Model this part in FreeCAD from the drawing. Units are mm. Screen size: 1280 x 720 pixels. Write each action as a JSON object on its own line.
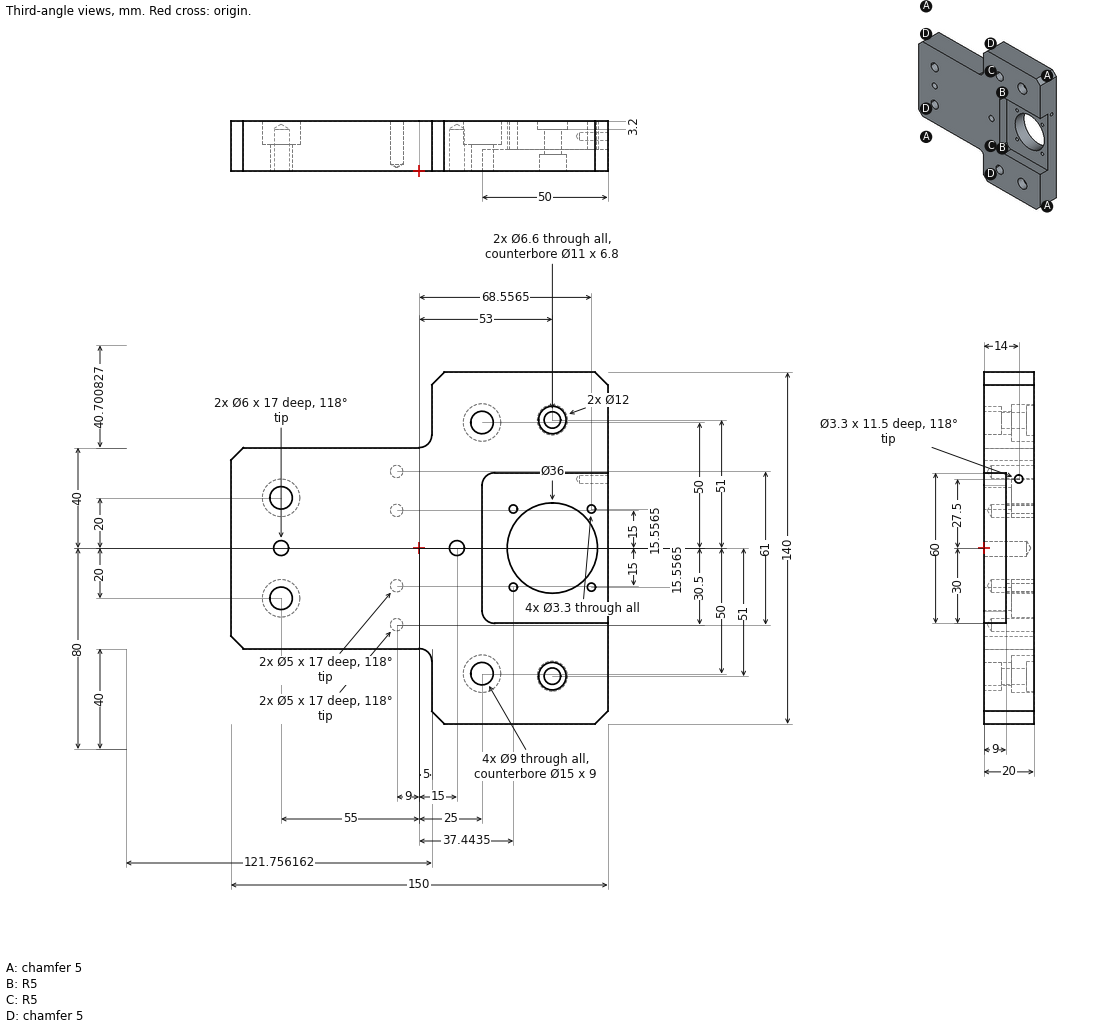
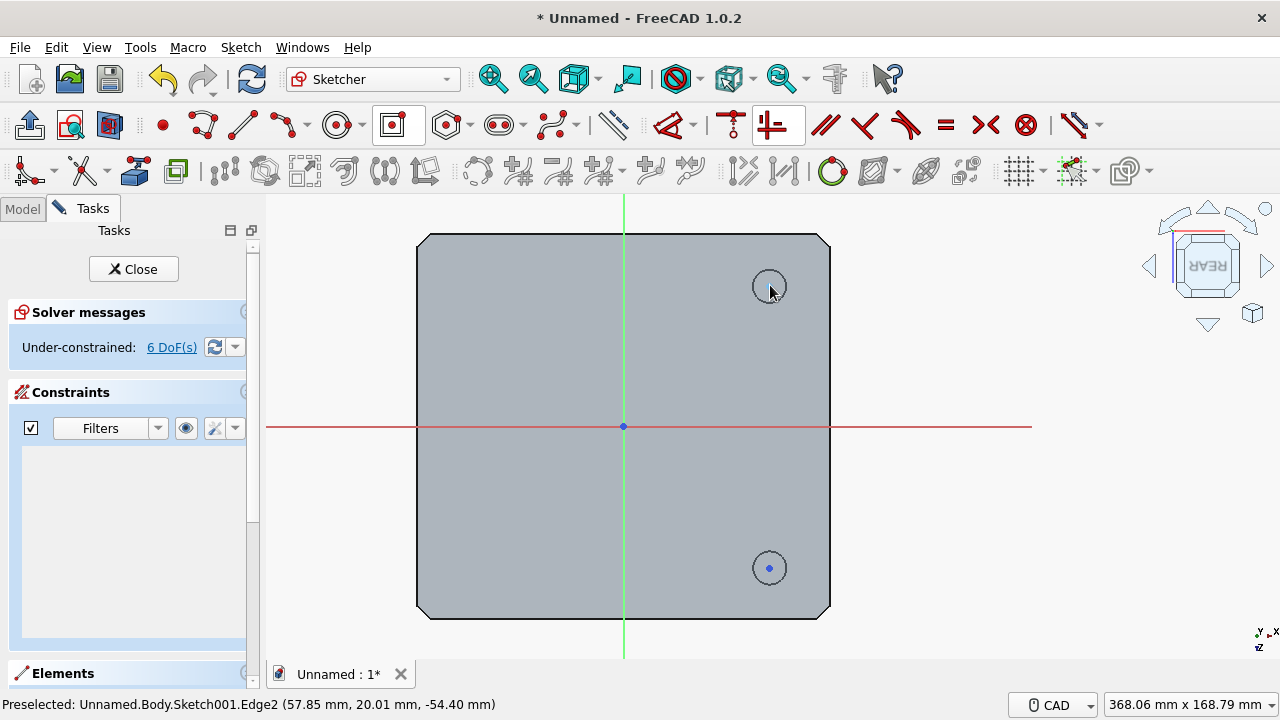
{"action": "left_click", "coordinate": [781, 556]}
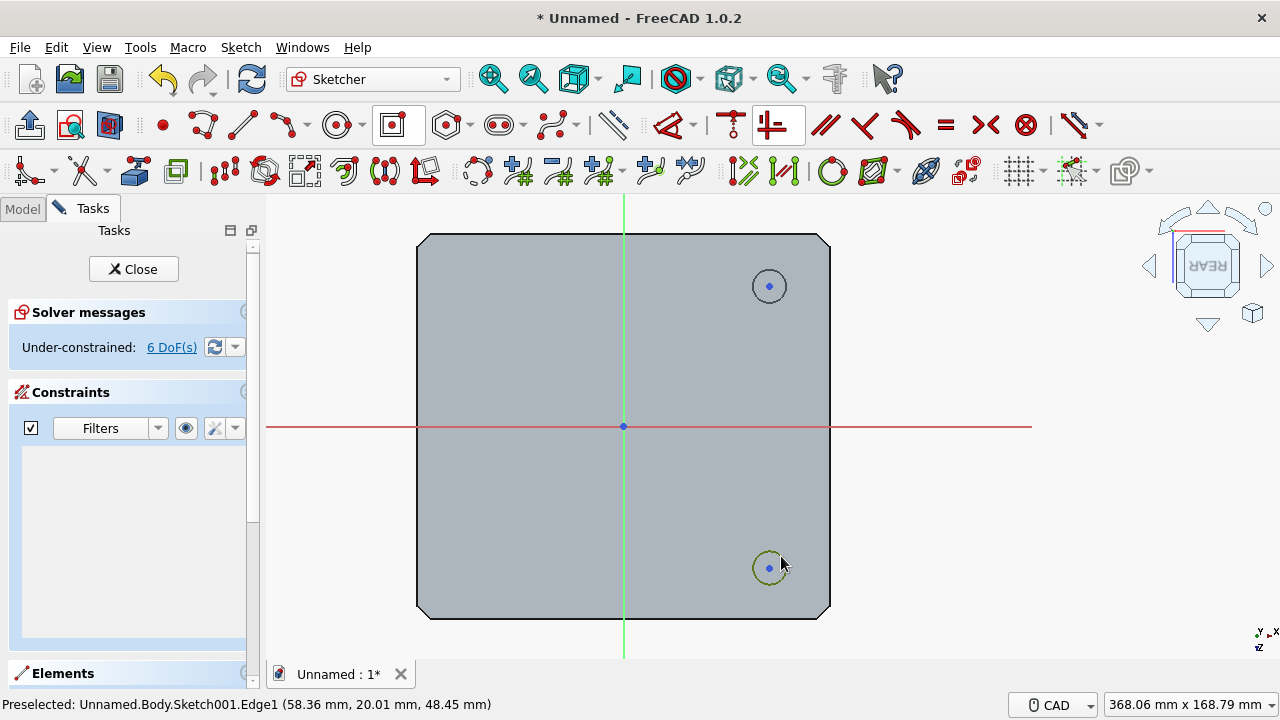
{"action": "left_click", "coordinate": [781, 275]}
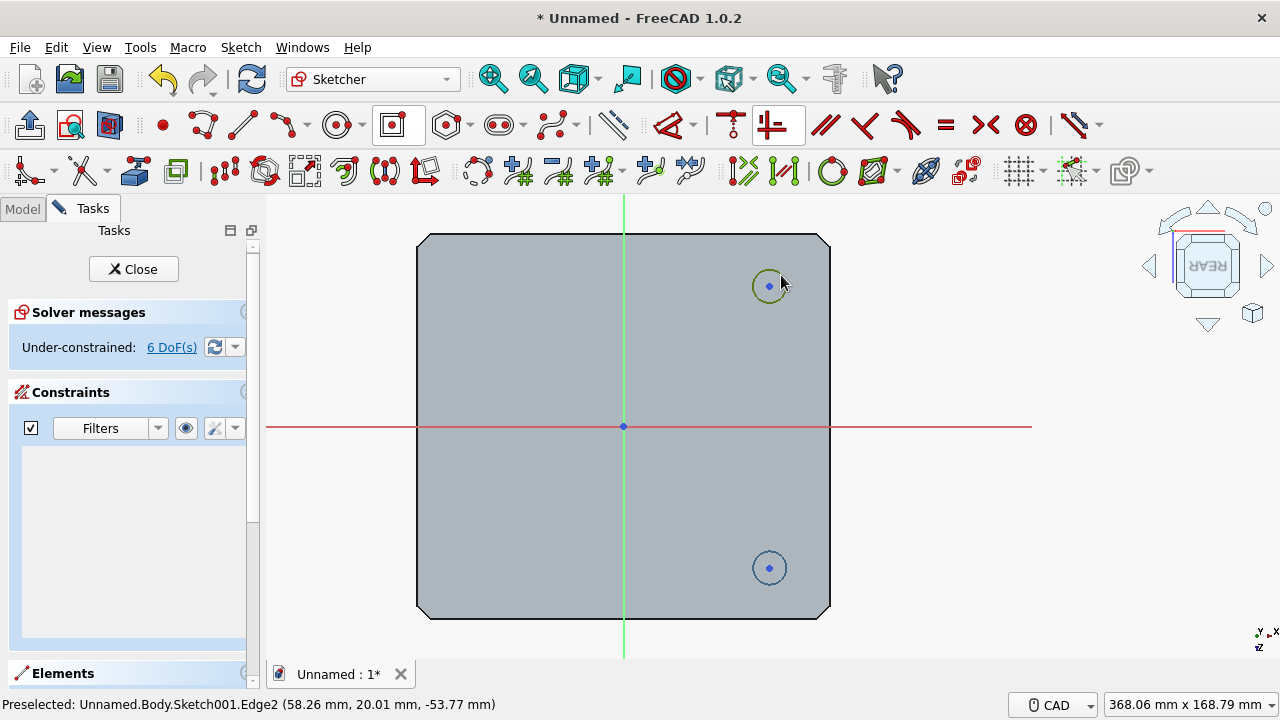
{"action": "left_click", "coordinate": [946, 126]}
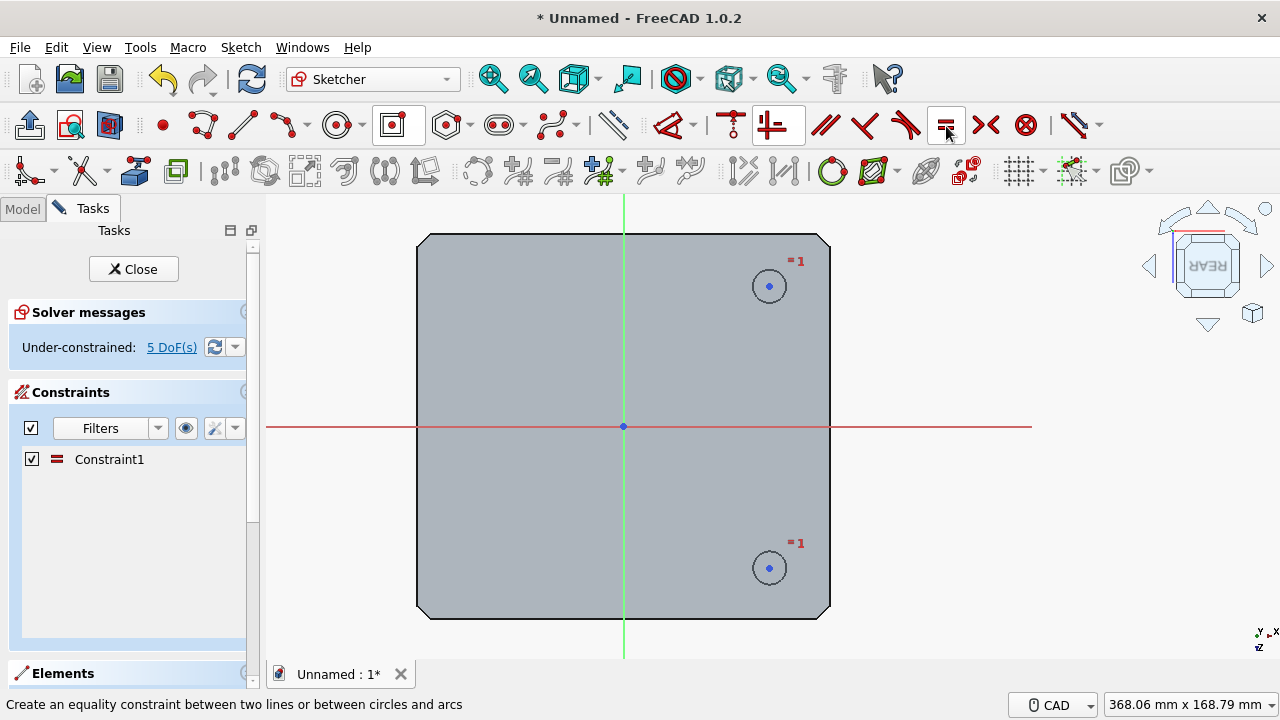
{"action": "left_click", "coordinate": [770, 568]}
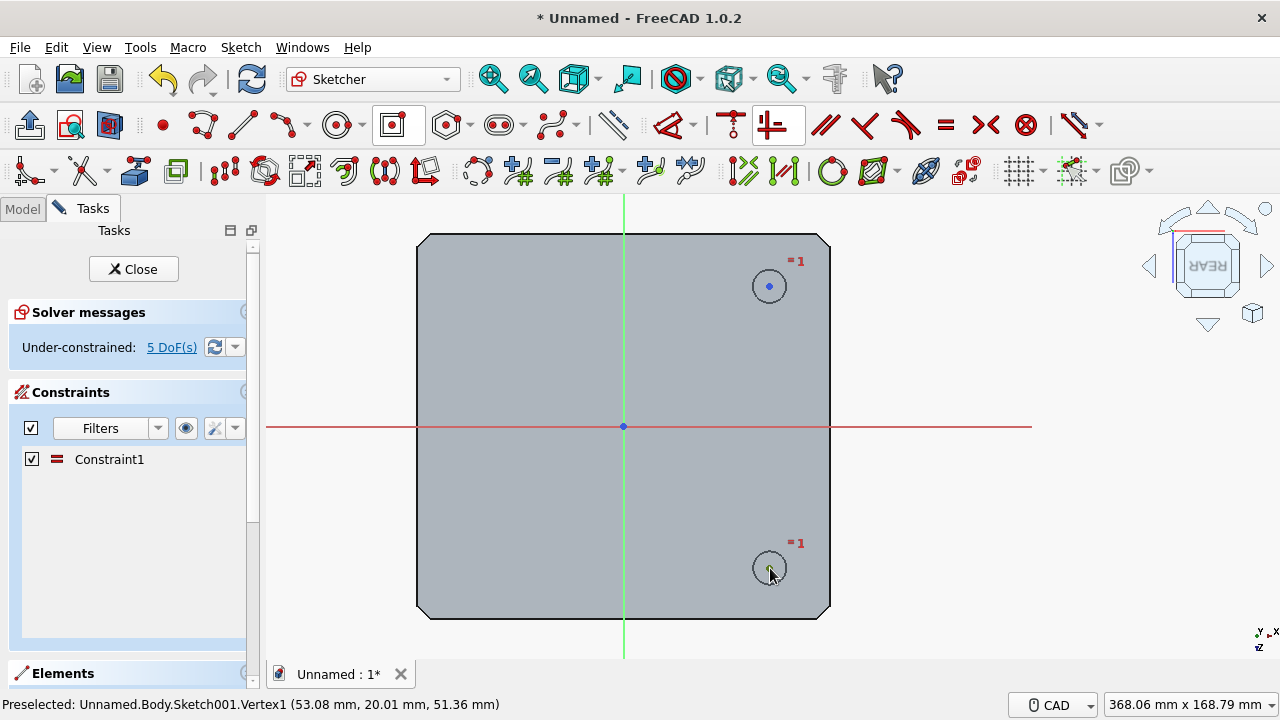
{"action": "left_click", "coordinate": [769, 286]}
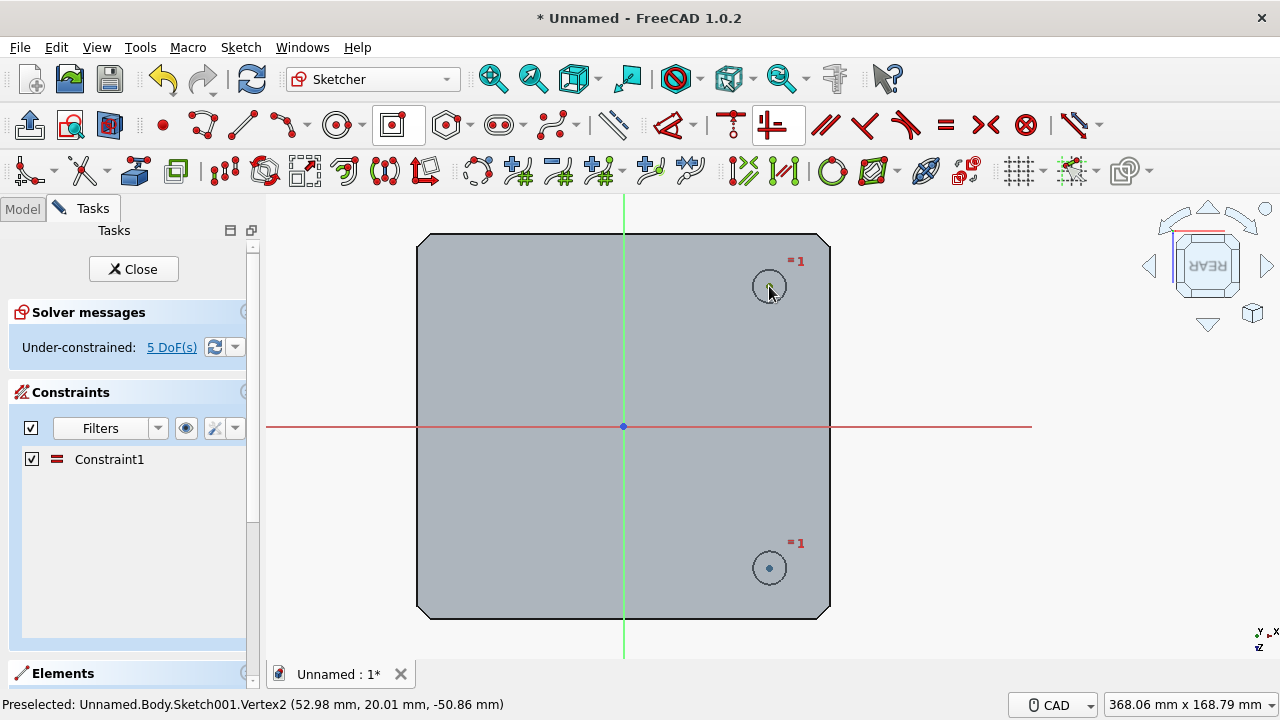
{"action": "left_click", "coordinate": [800, 126]}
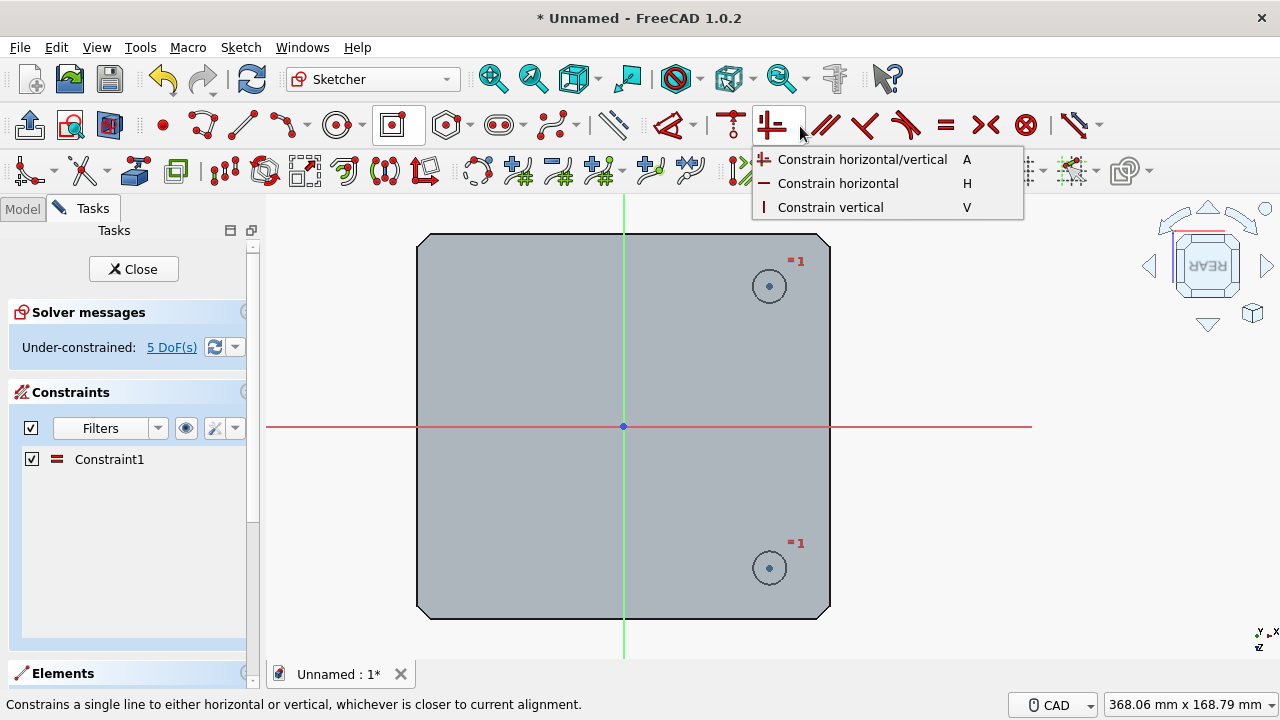
{"action": "left_click", "coordinate": [888, 207]}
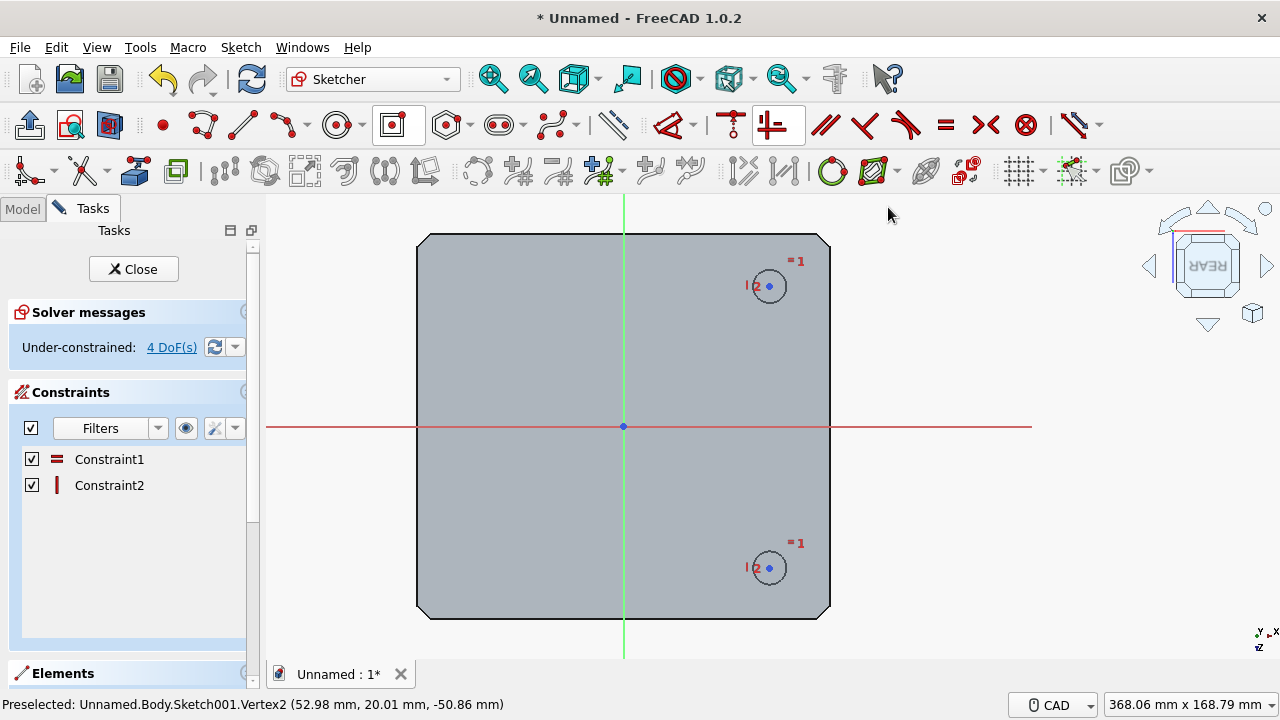
{"action": "left_click", "coordinate": [668, 126]}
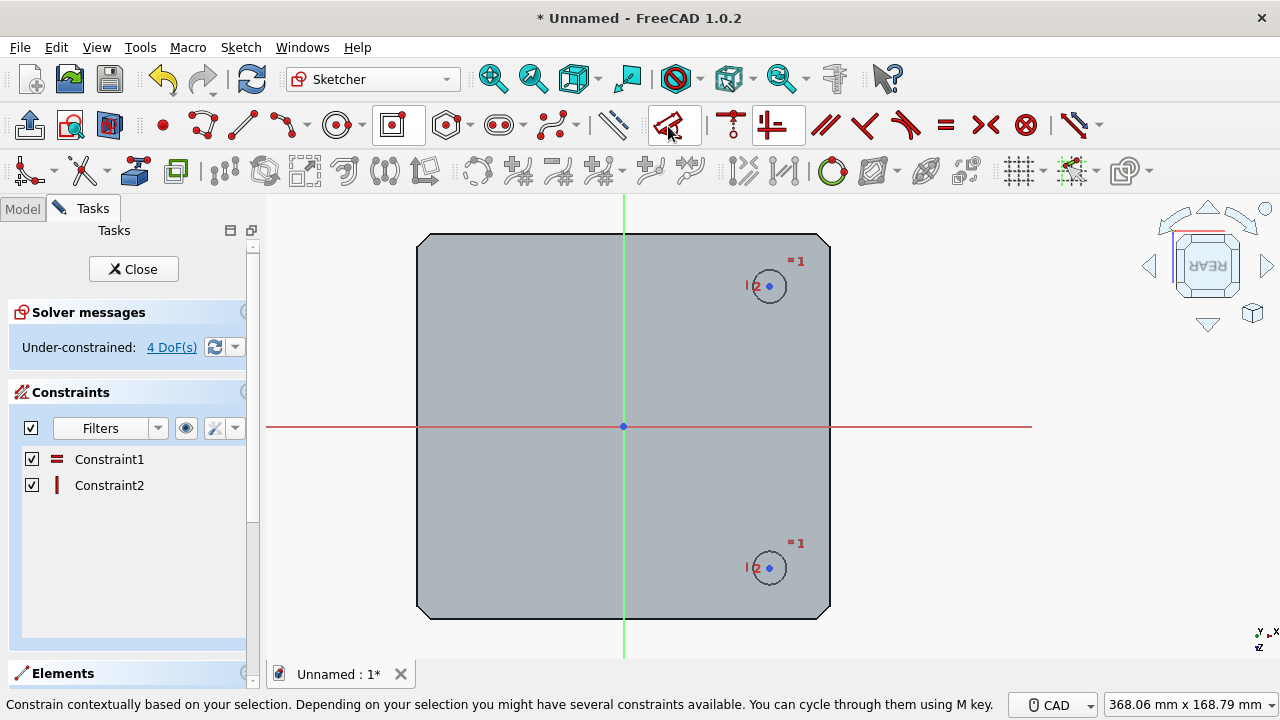
{"action": "left_click", "coordinate": [781, 556]}
{"action": "left_click", "coordinate": [803, 533]}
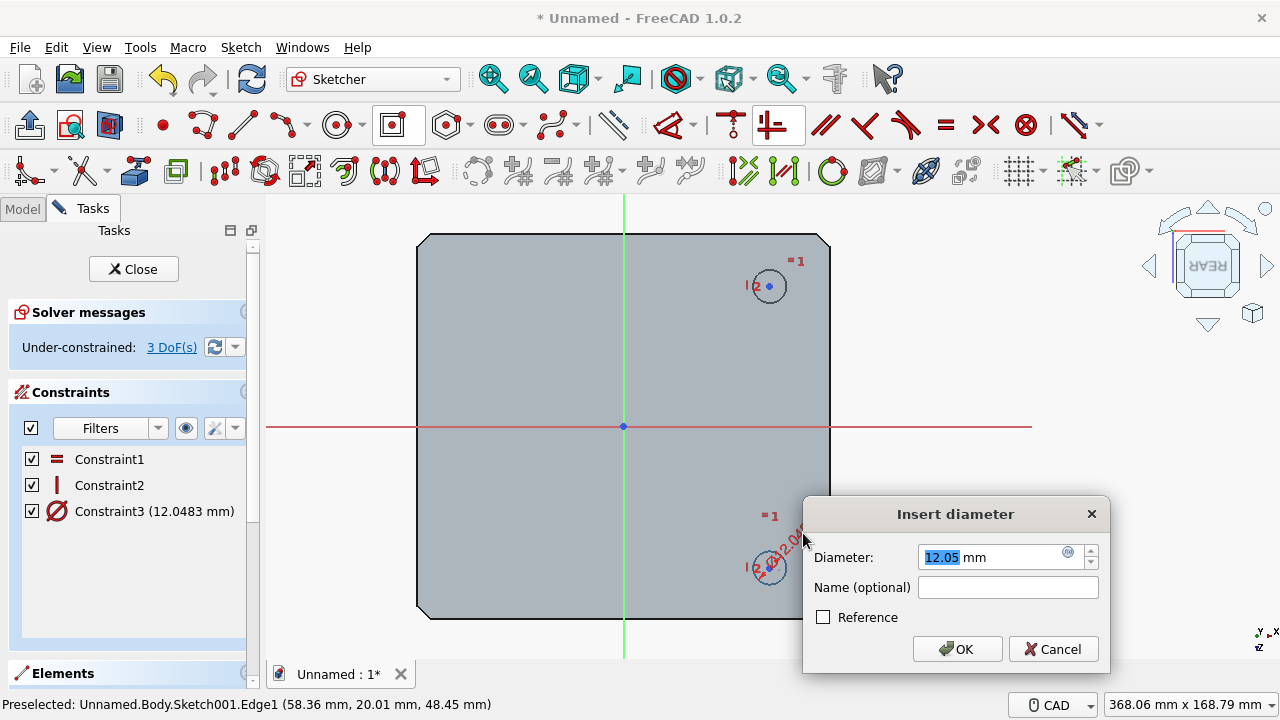
{"action": "type", "text": "12"}
{"action": "key", "text": "Return"}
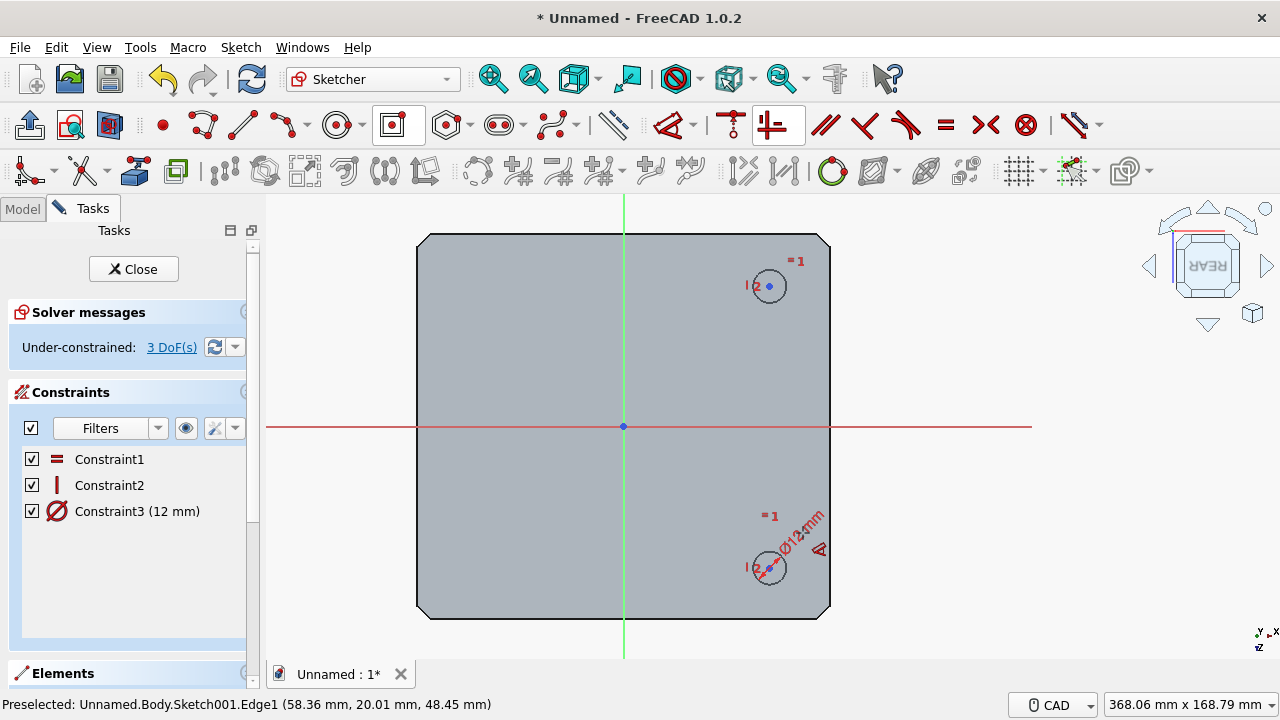
{"action": "left_click", "coordinate": [770, 568]}
{"action": "left_click", "coordinate": [697, 602]}